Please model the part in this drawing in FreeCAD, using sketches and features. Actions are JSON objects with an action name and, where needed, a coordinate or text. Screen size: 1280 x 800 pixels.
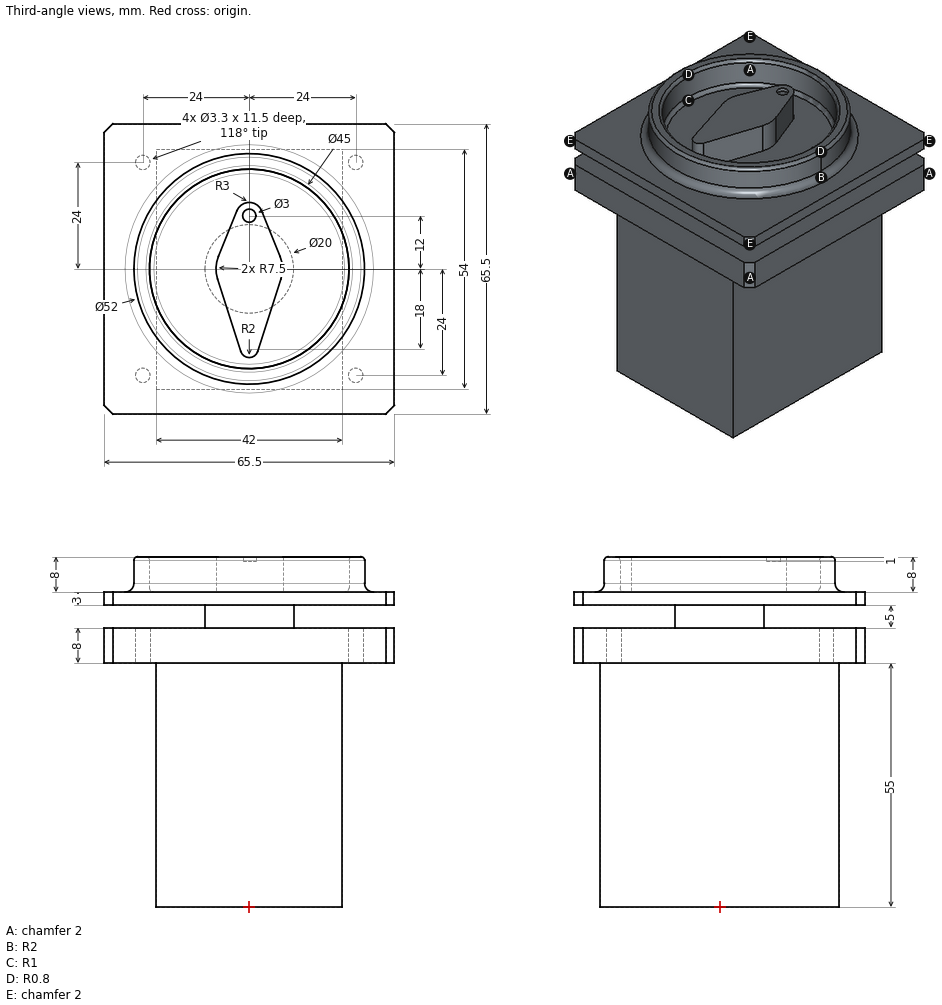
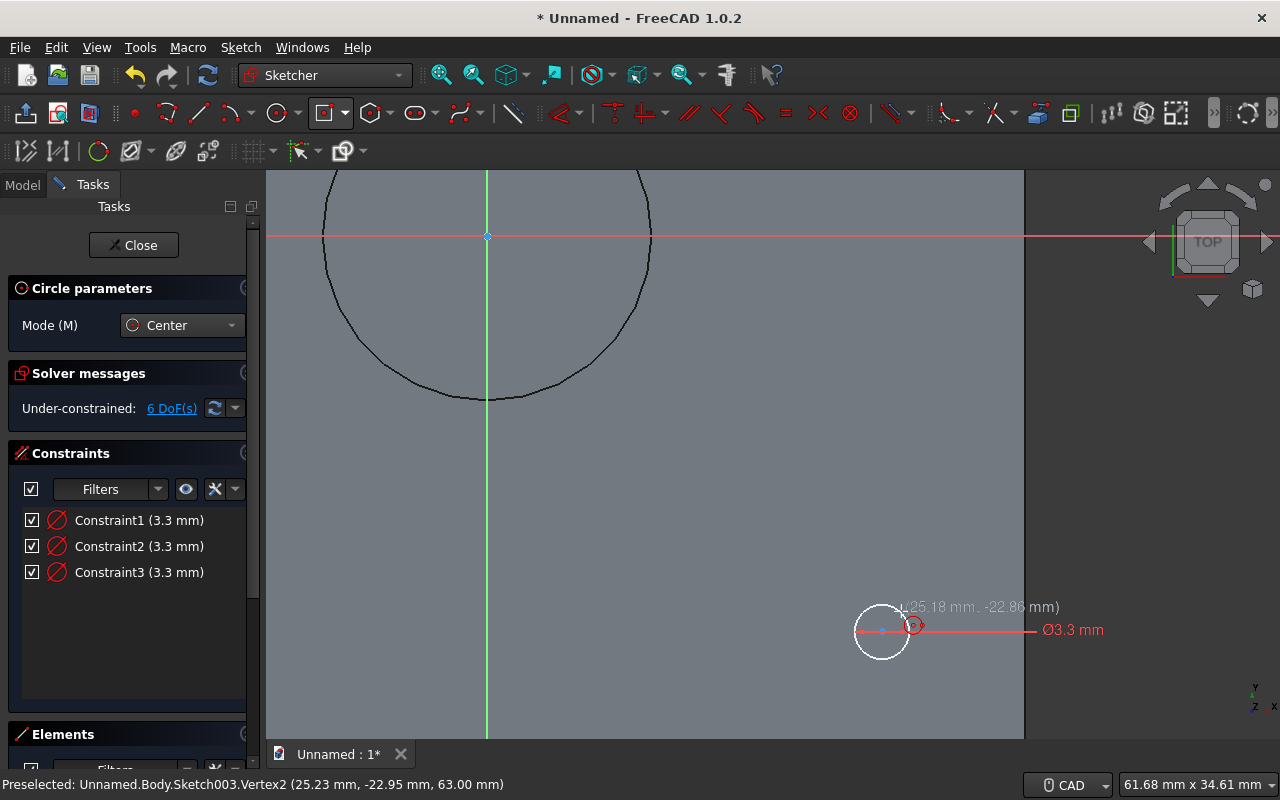
{"action": "scroll", "coordinate": [882, 633], "scroll_direction": "down", "scroll_amount": 4}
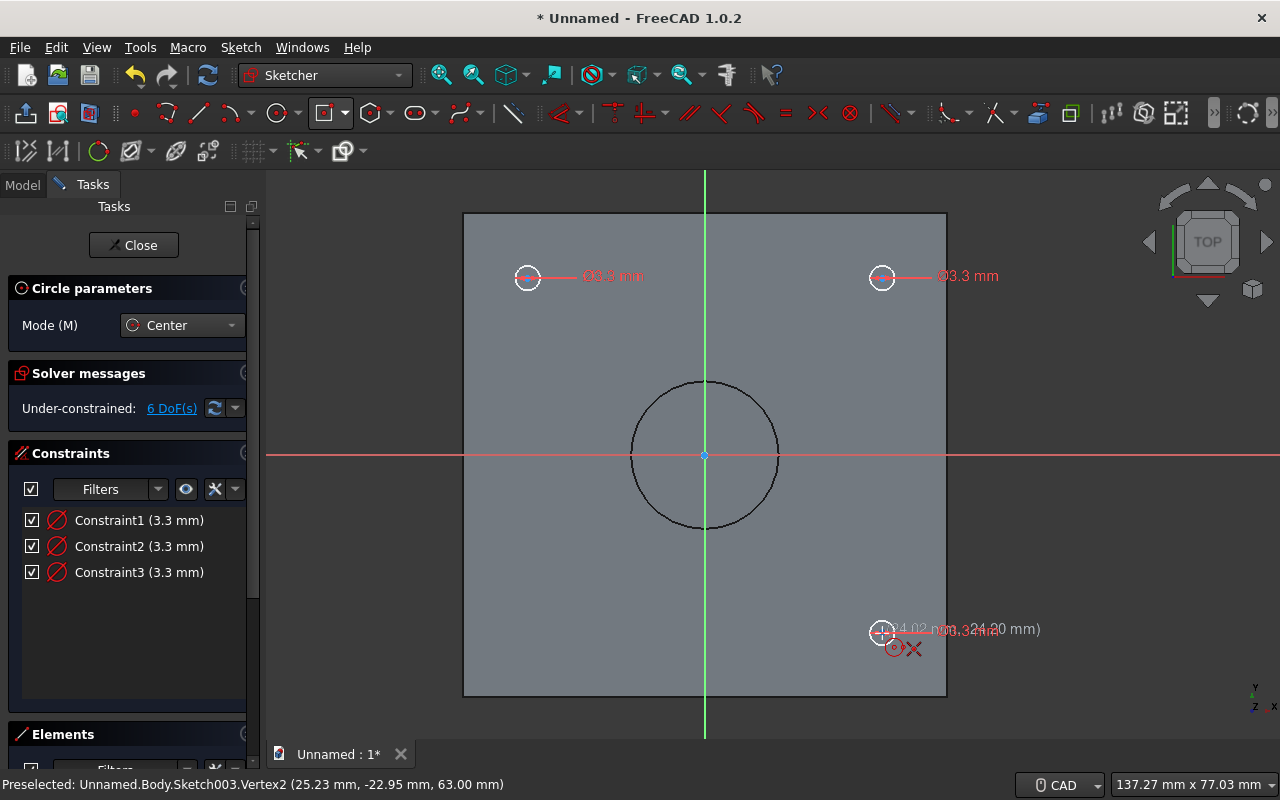
{"action": "scroll", "coordinate": [528, 632], "scroll_direction": "up", "scroll_amount": 4}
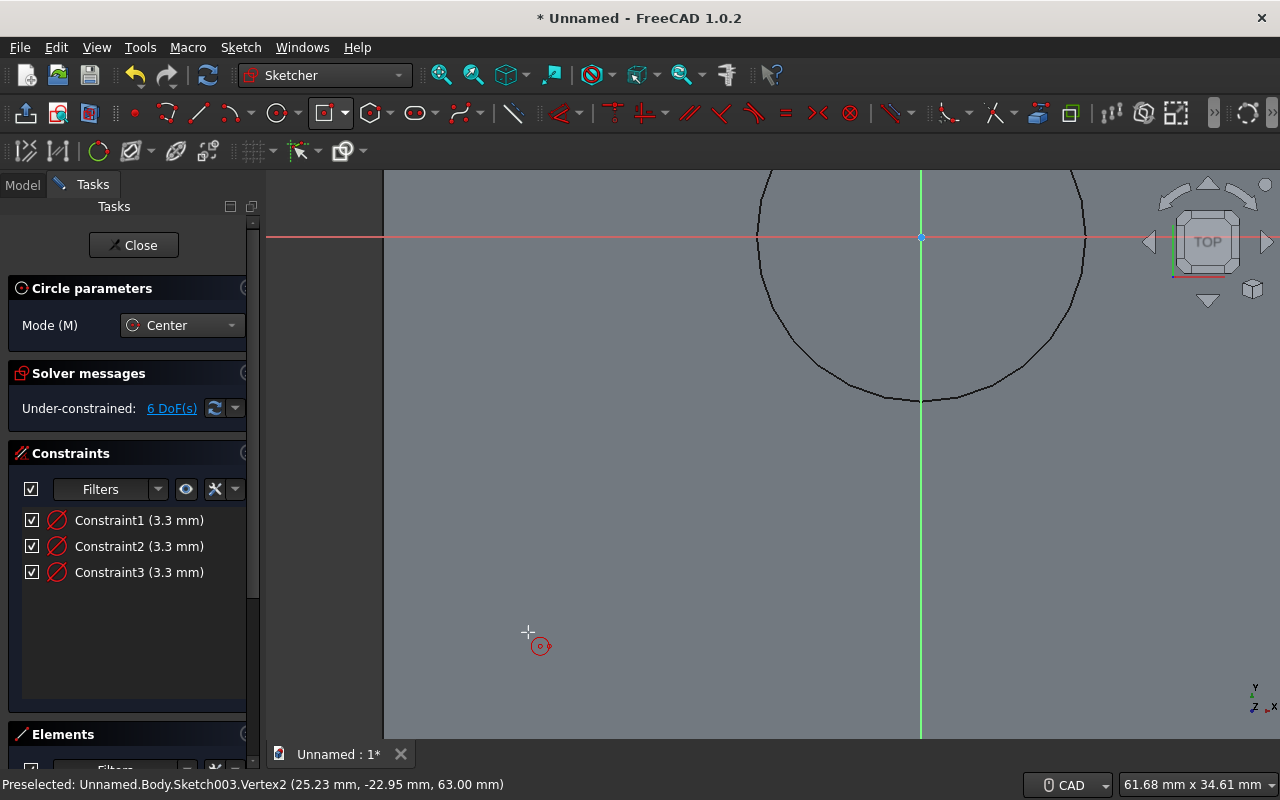
{"action": "left_click", "coordinate": [527, 632]}
{"action": "mouse_move", "coordinate": [546, 613]}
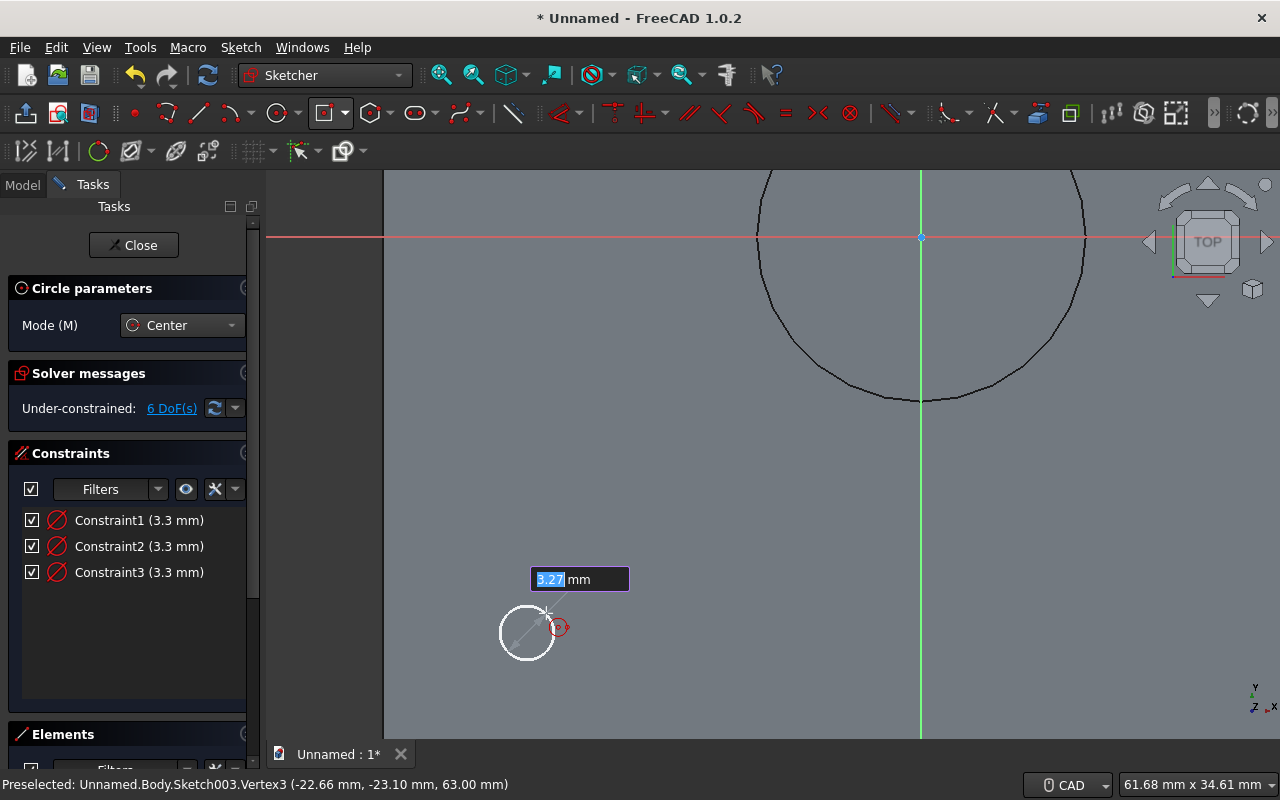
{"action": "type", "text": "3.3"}
{"action": "key", "text": "Return"}
{"action": "key", "text": "Escape"}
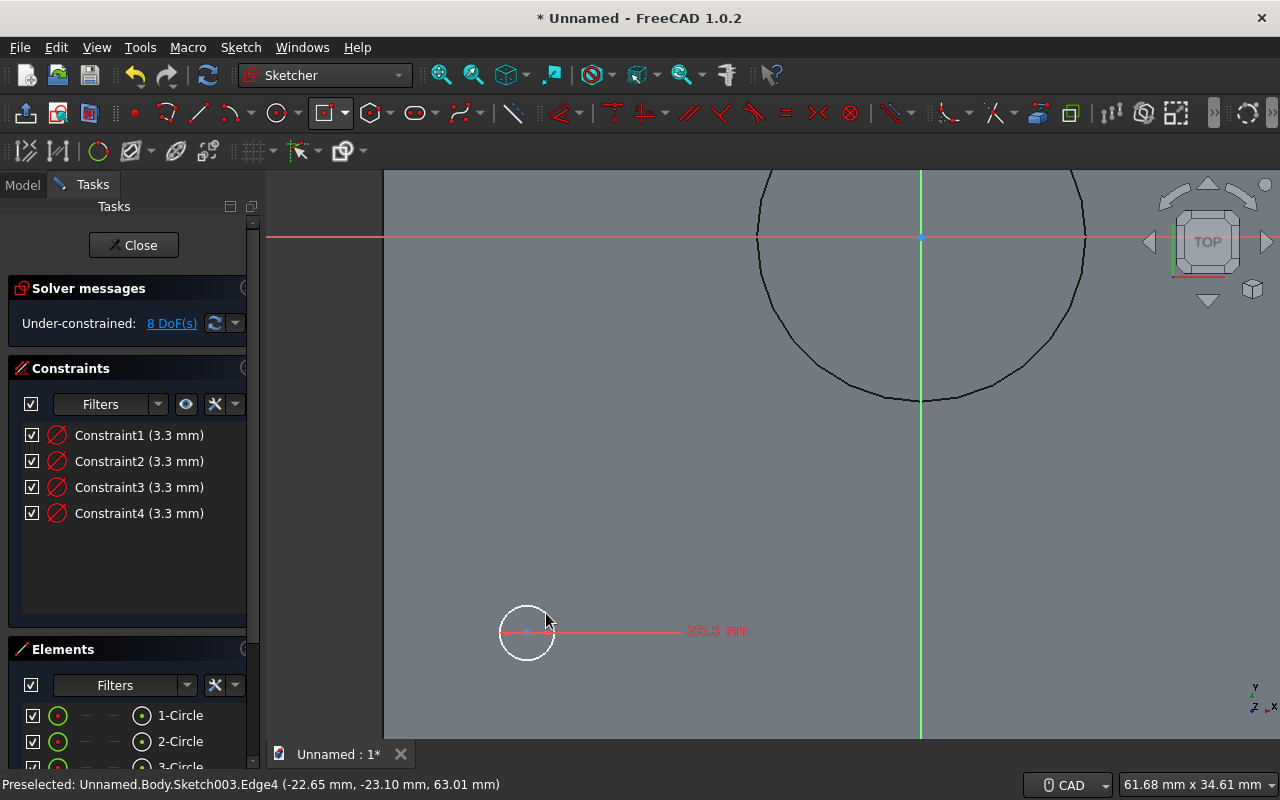
{"action": "scroll", "coordinate": [528, 632], "scroll_direction": "down", "scroll_amount": 4}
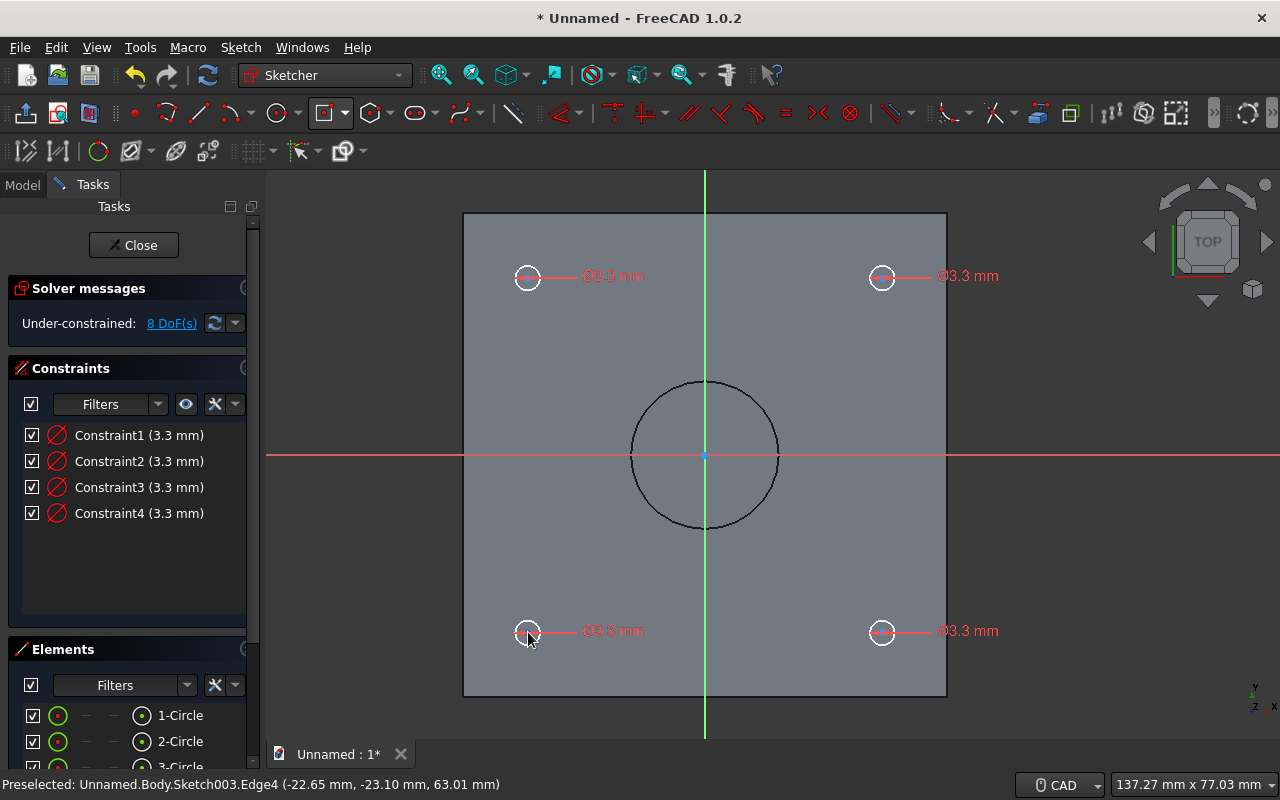
{"action": "left_click", "coordinate": [528, 278]}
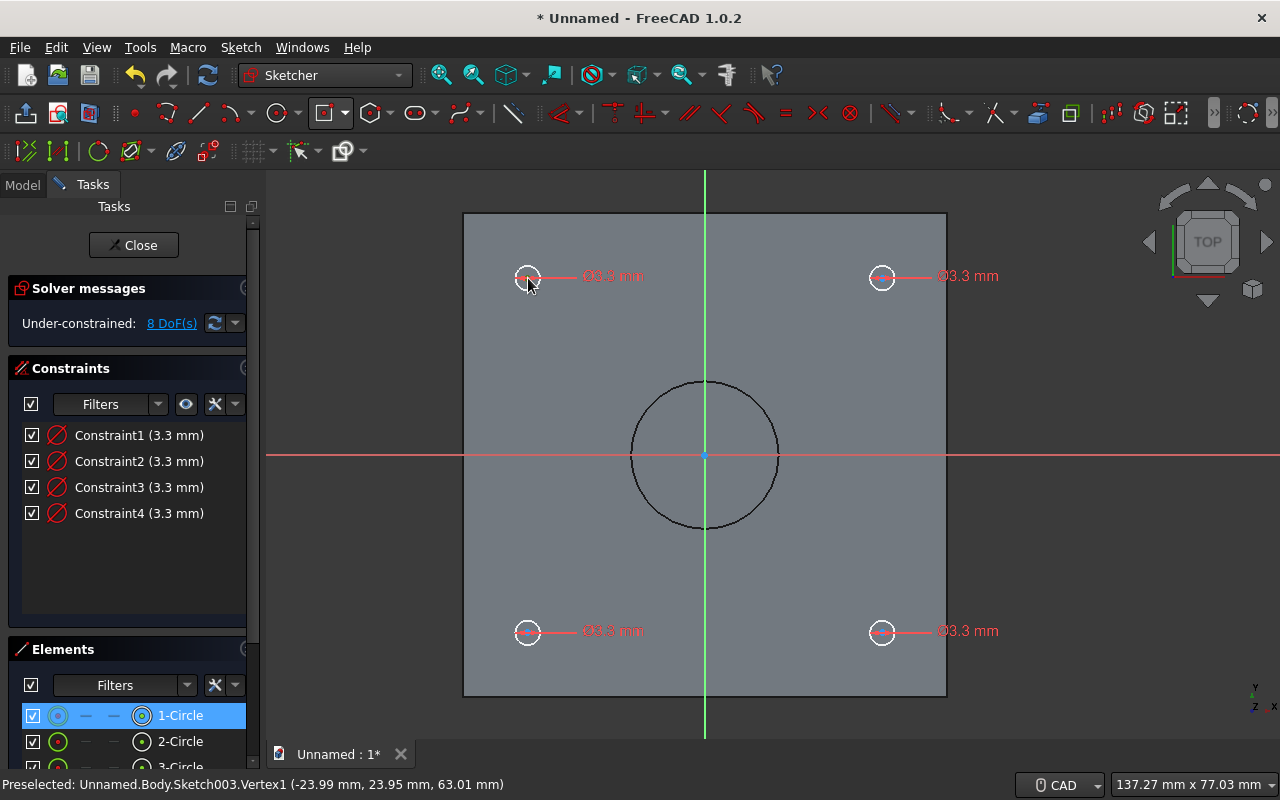
{"action": "left_click", "coordinate": [882, 278]}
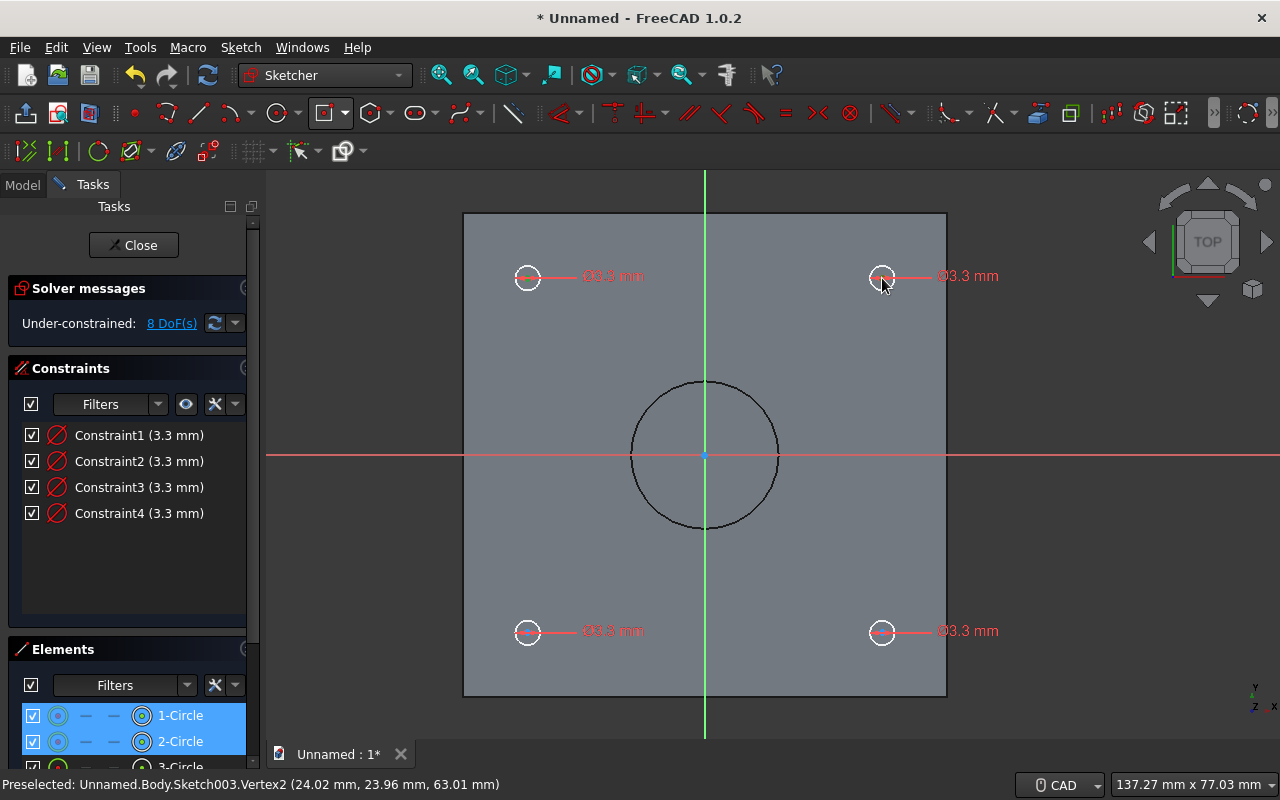
{"action": "key", "text": "h"}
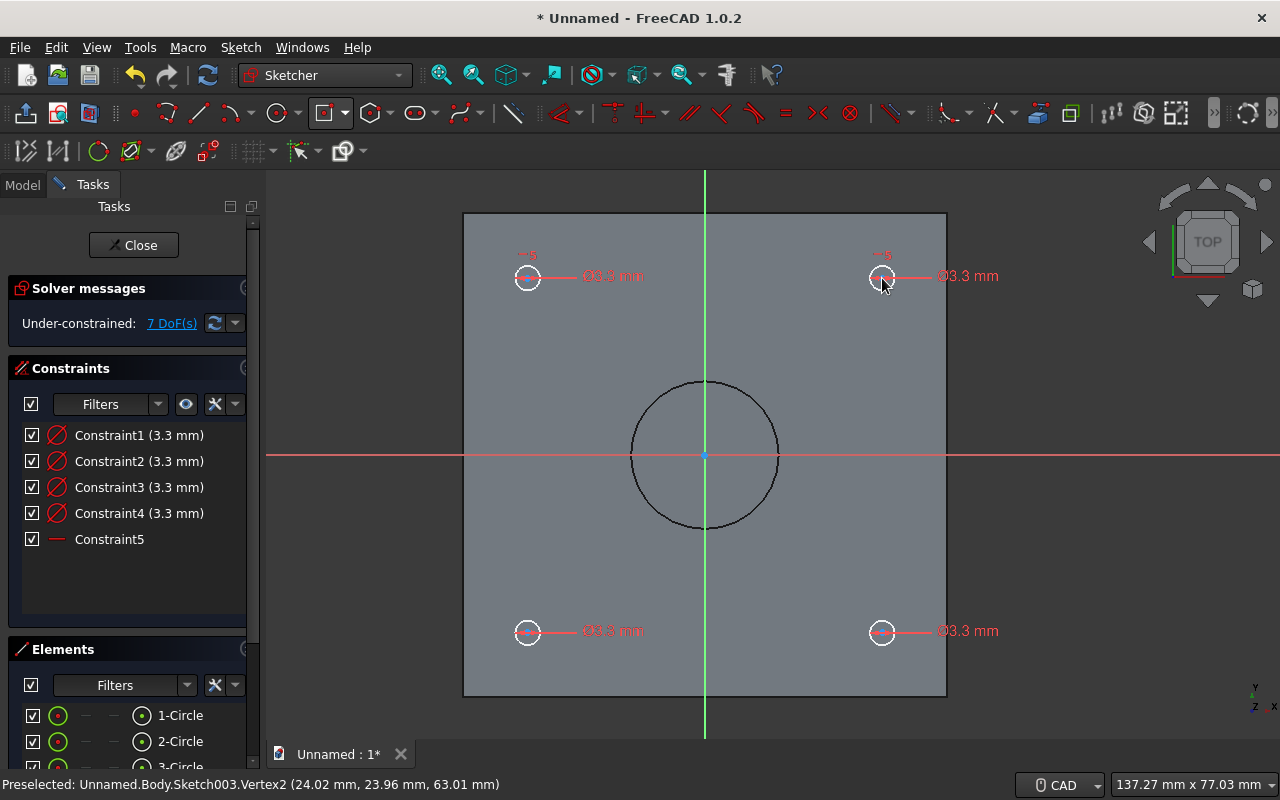
{"action": "left_click", "coordinate": [882, 278]}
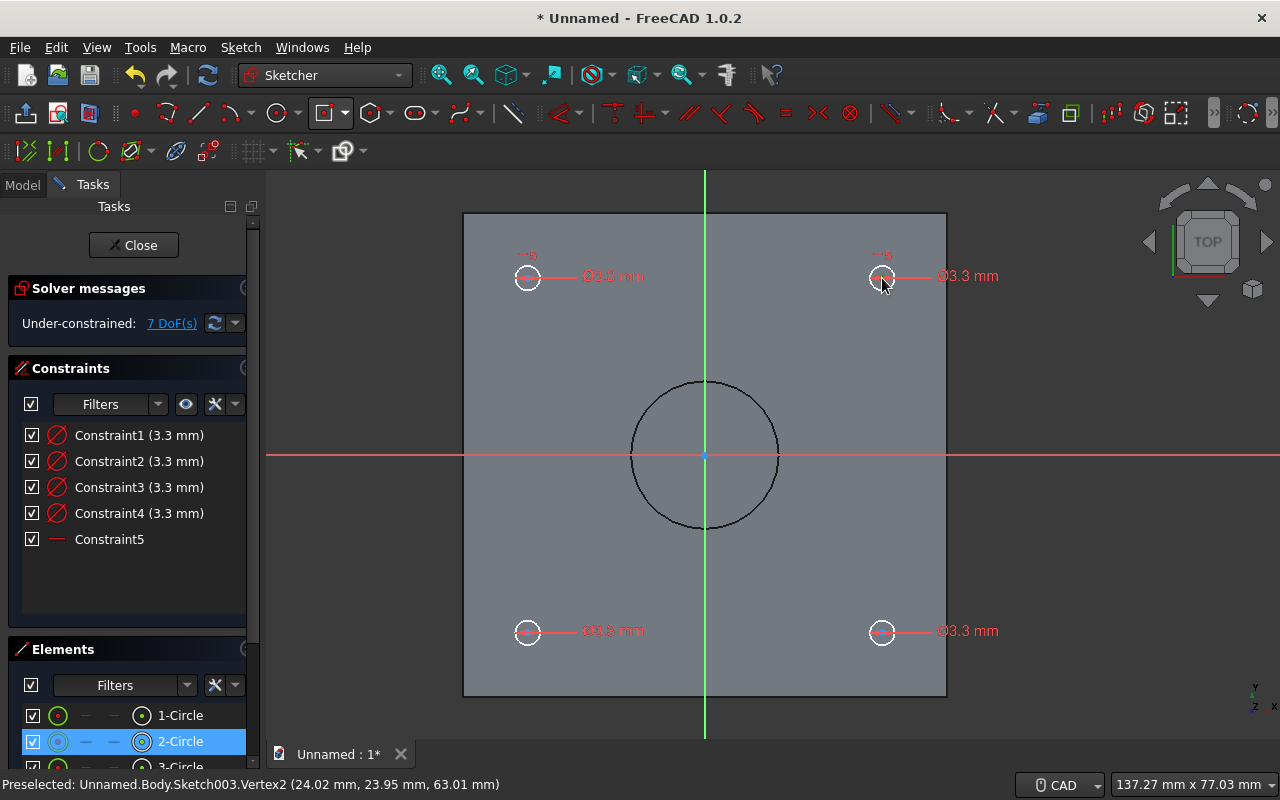
{"action": "left_click", "coordinate": [882, 633]}